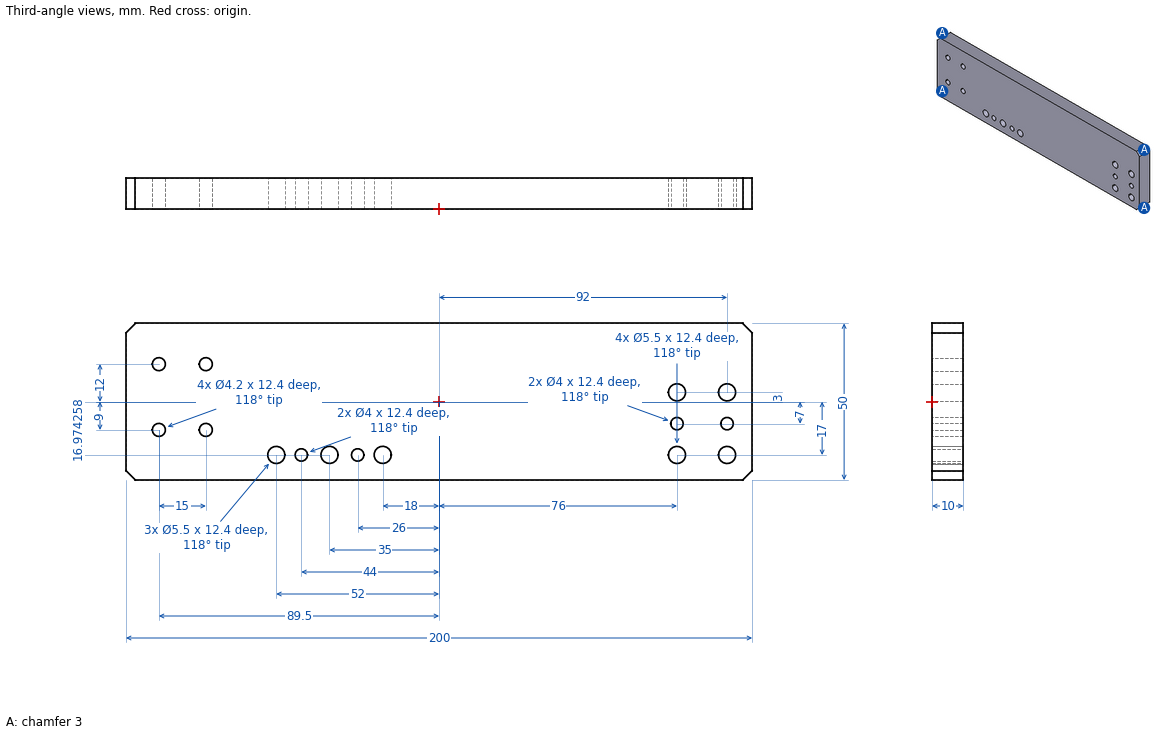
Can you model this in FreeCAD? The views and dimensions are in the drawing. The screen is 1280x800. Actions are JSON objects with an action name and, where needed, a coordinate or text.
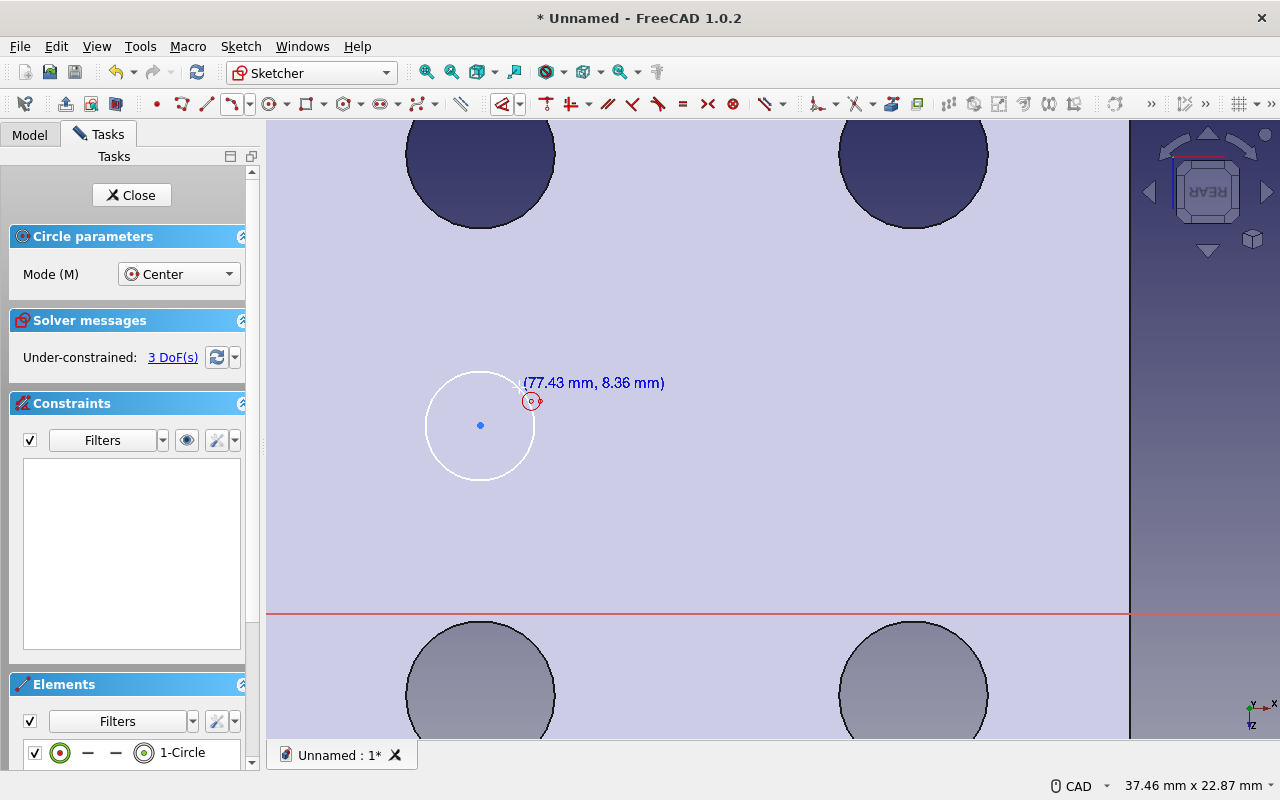
{"action": "left_click", "coordinate": [913, 425]}
{"action": "left_click", "coordinate": [952, 387]}
{"action": "key", "text": "Escape"}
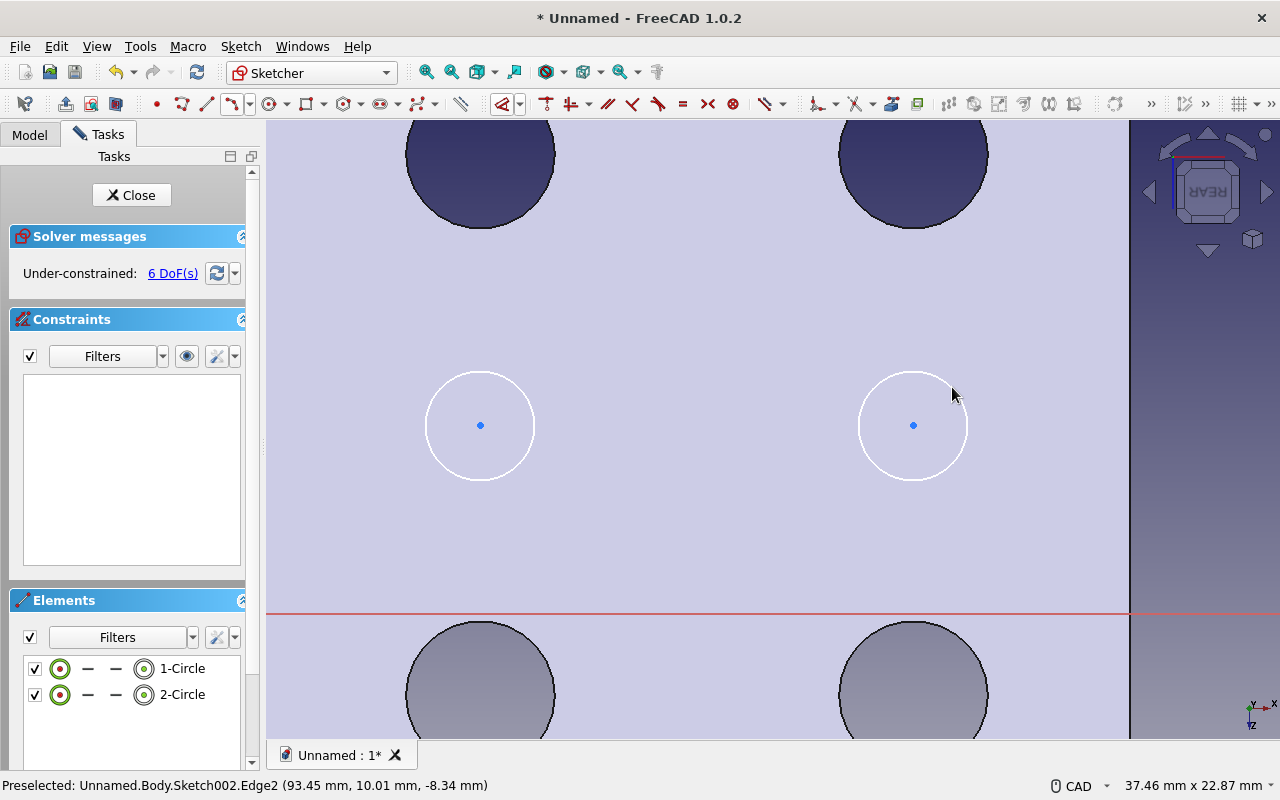
{"action": "left_click", "coordinate": [518, 387]}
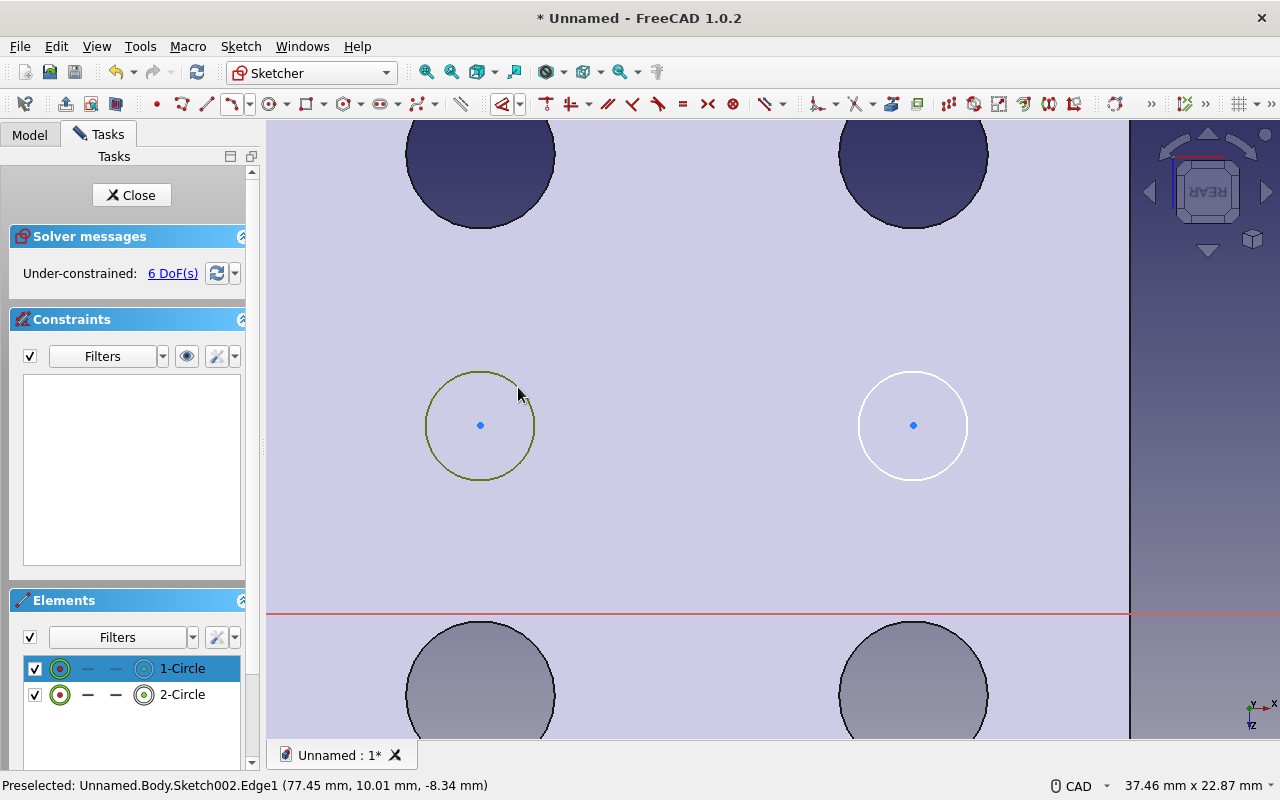
{"action": "left_click", "coordinate": [951, 387]}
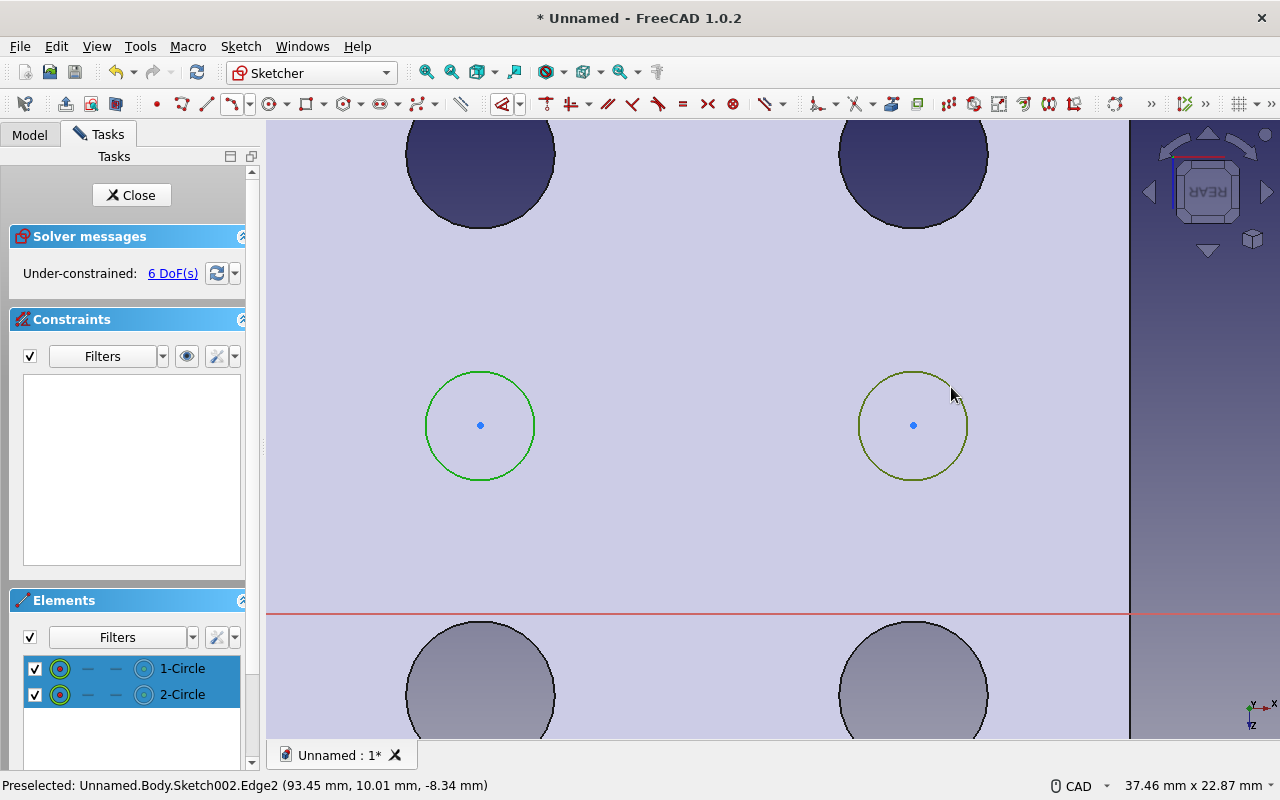
{"action": "left_click", "coordinate": [683, 104]}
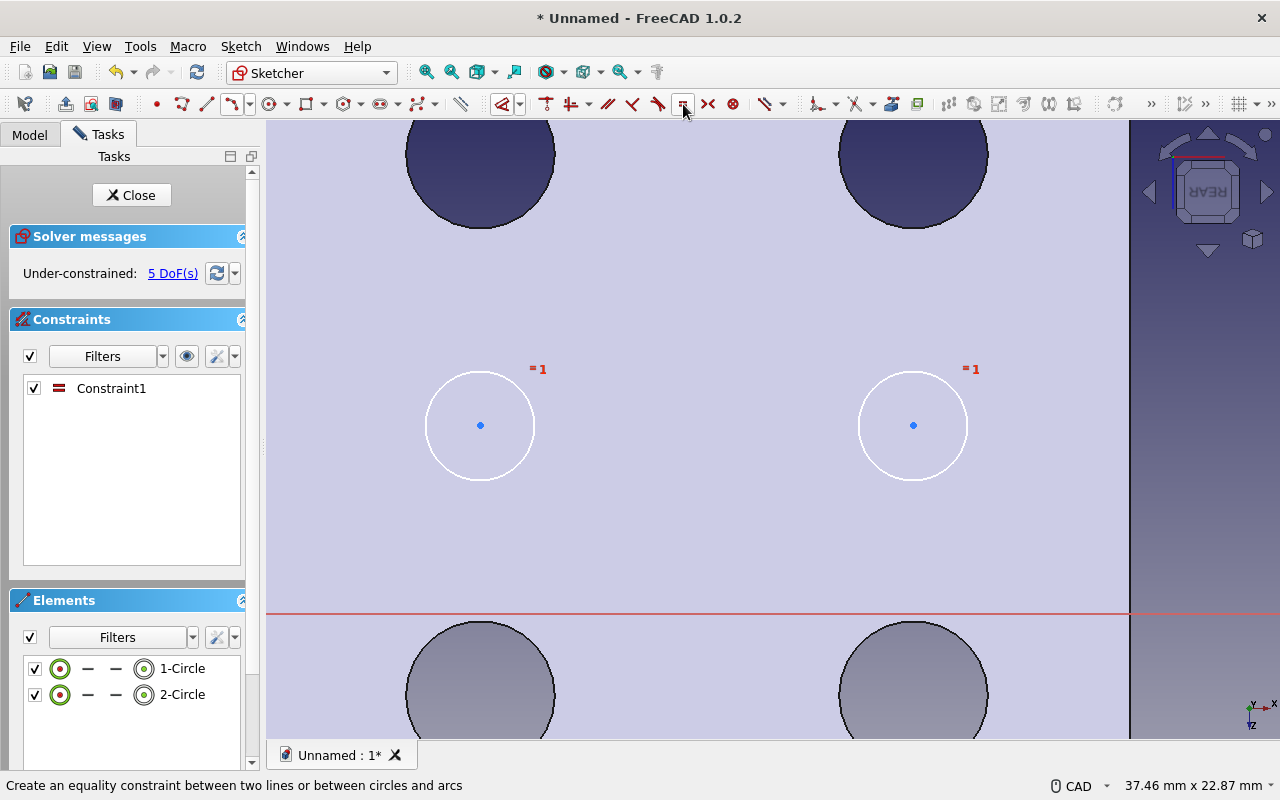
{"action": "left_click", "coordinate": [480, 426]}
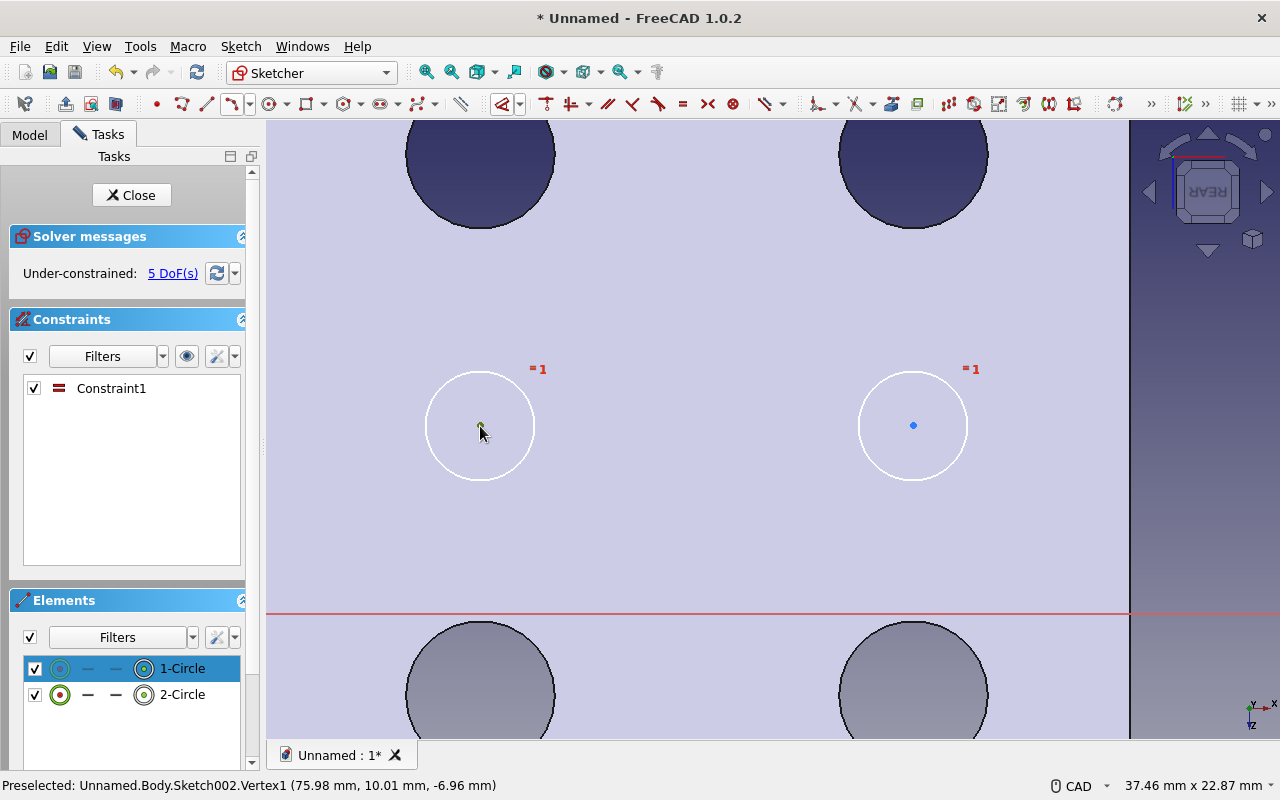
{"action": "left_click", "coordinate": [913, 426]}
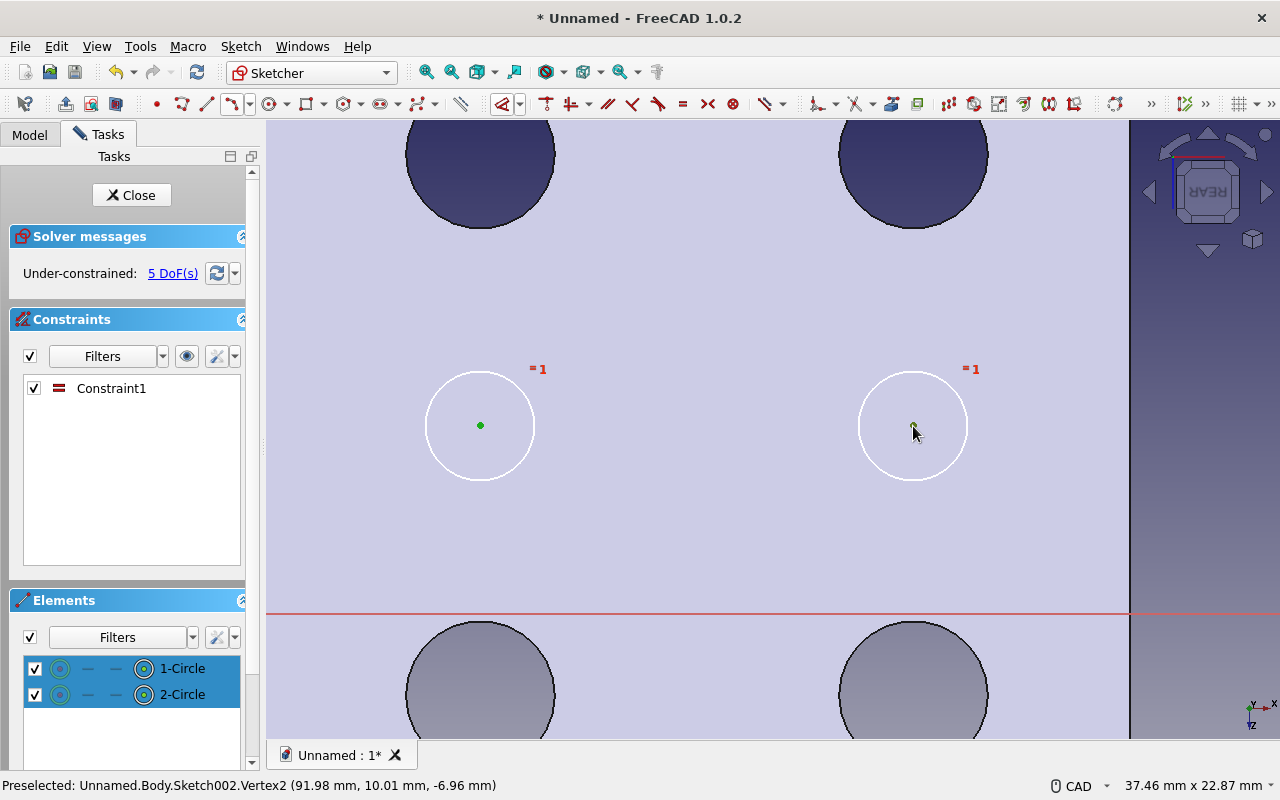
{"action": "key", "text": "h"}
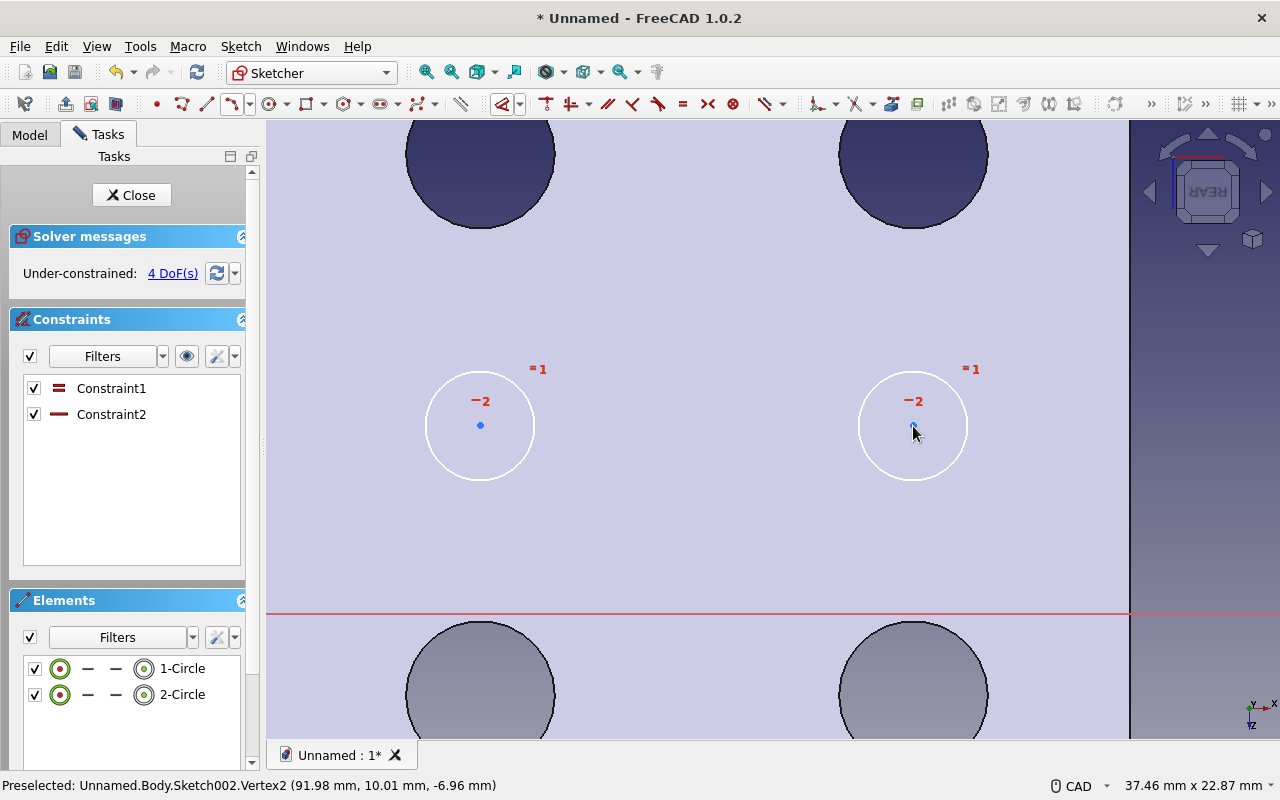
{"action": "key", "text": "d"}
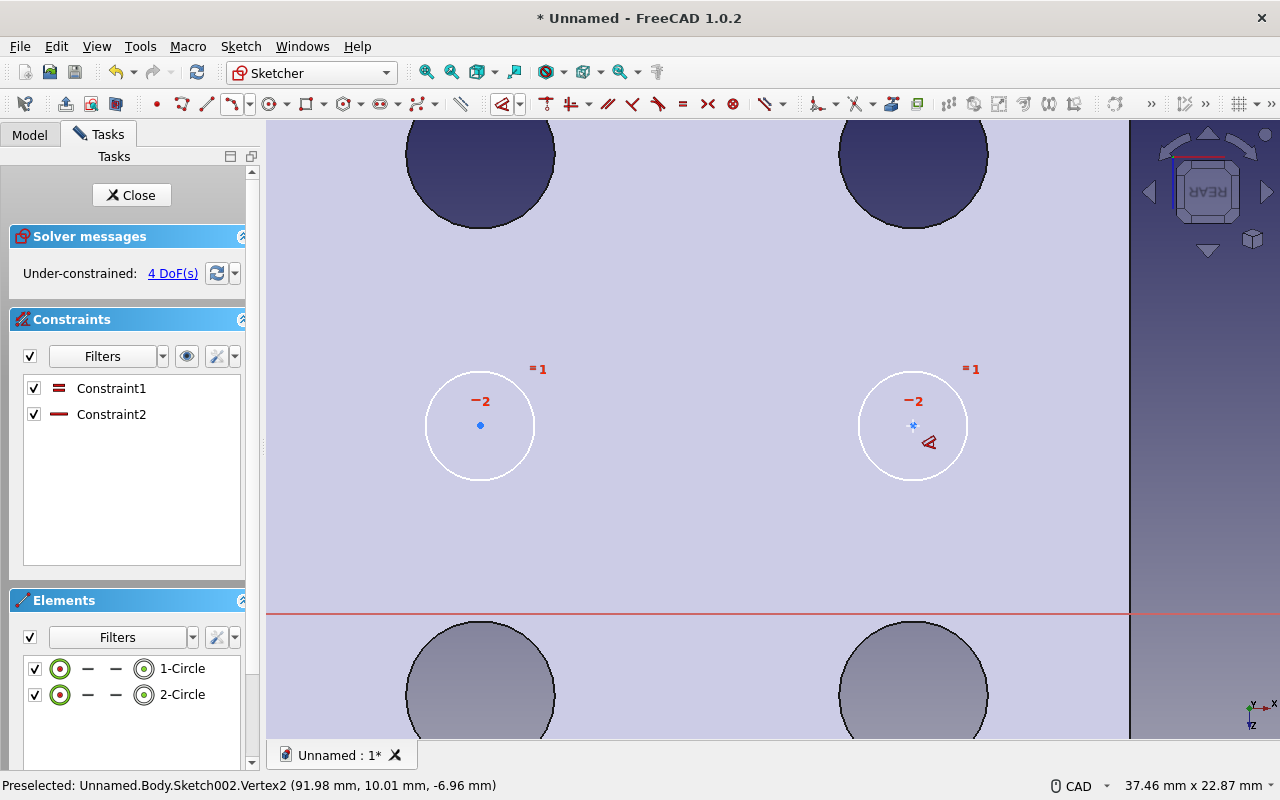
{"action": "left_click", "coordinate": [518, 387]}
{"action": "left_click", "coordinate": [540, 364]}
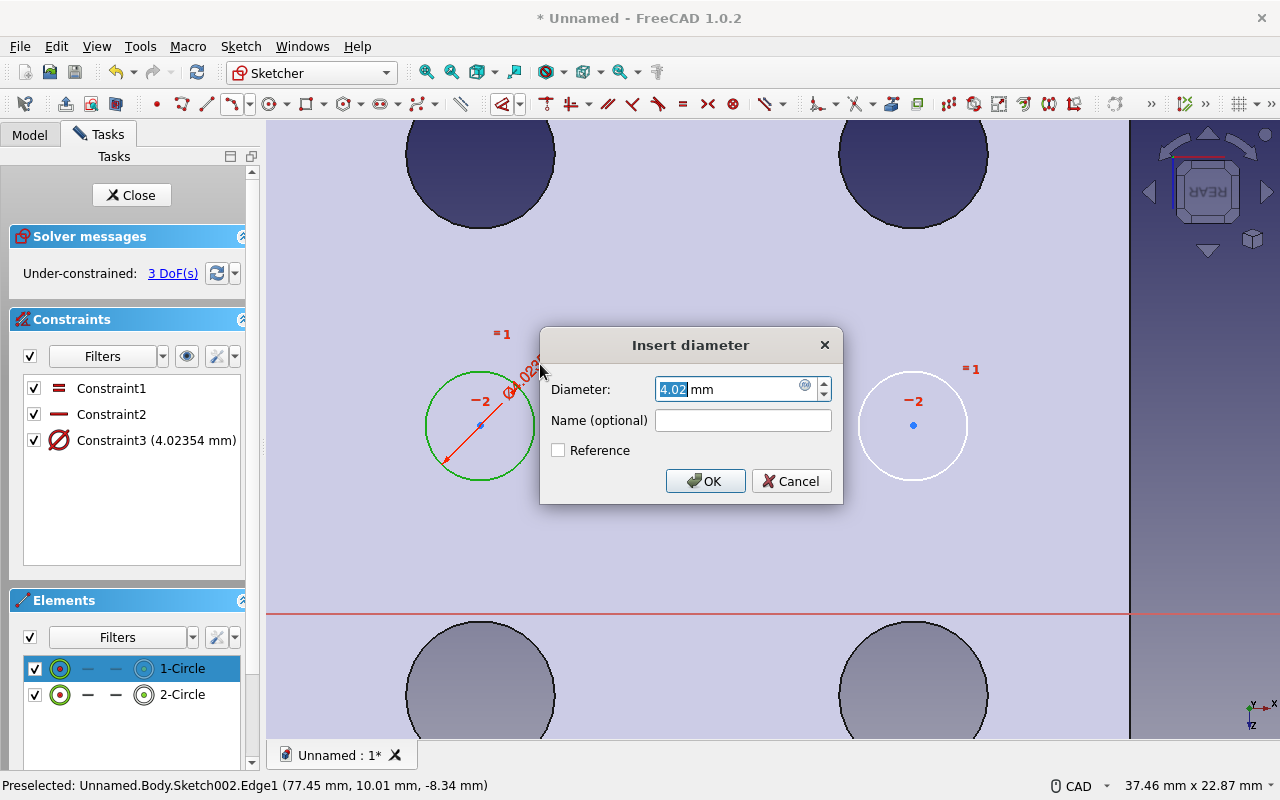
{"action": "type", "text": "4"}
{"action": "key", "text": "Return"}